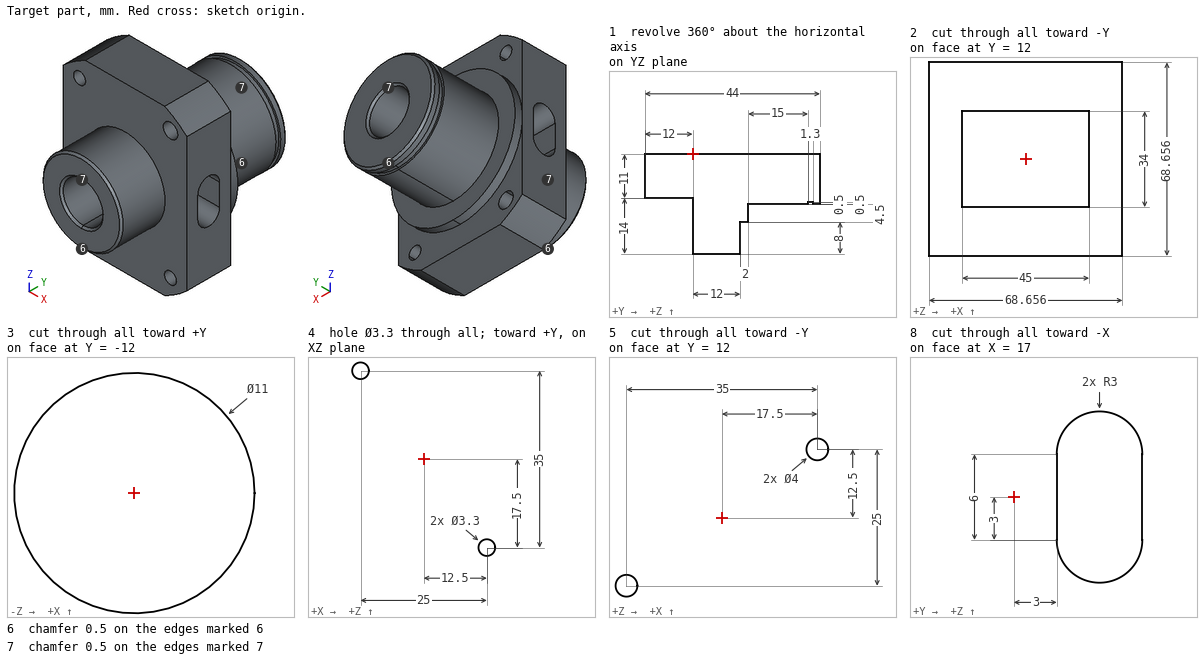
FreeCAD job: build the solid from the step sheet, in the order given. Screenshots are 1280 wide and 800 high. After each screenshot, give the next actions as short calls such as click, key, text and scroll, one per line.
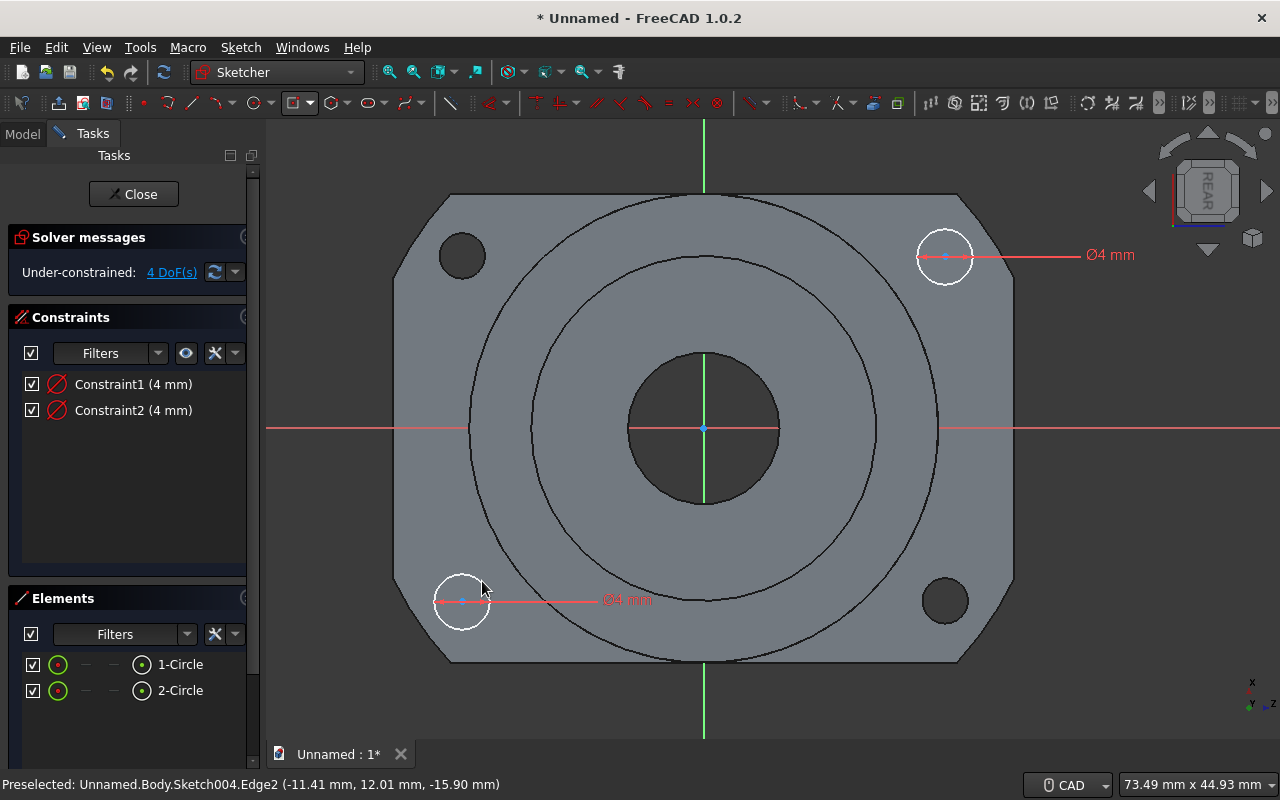
click(490, 104)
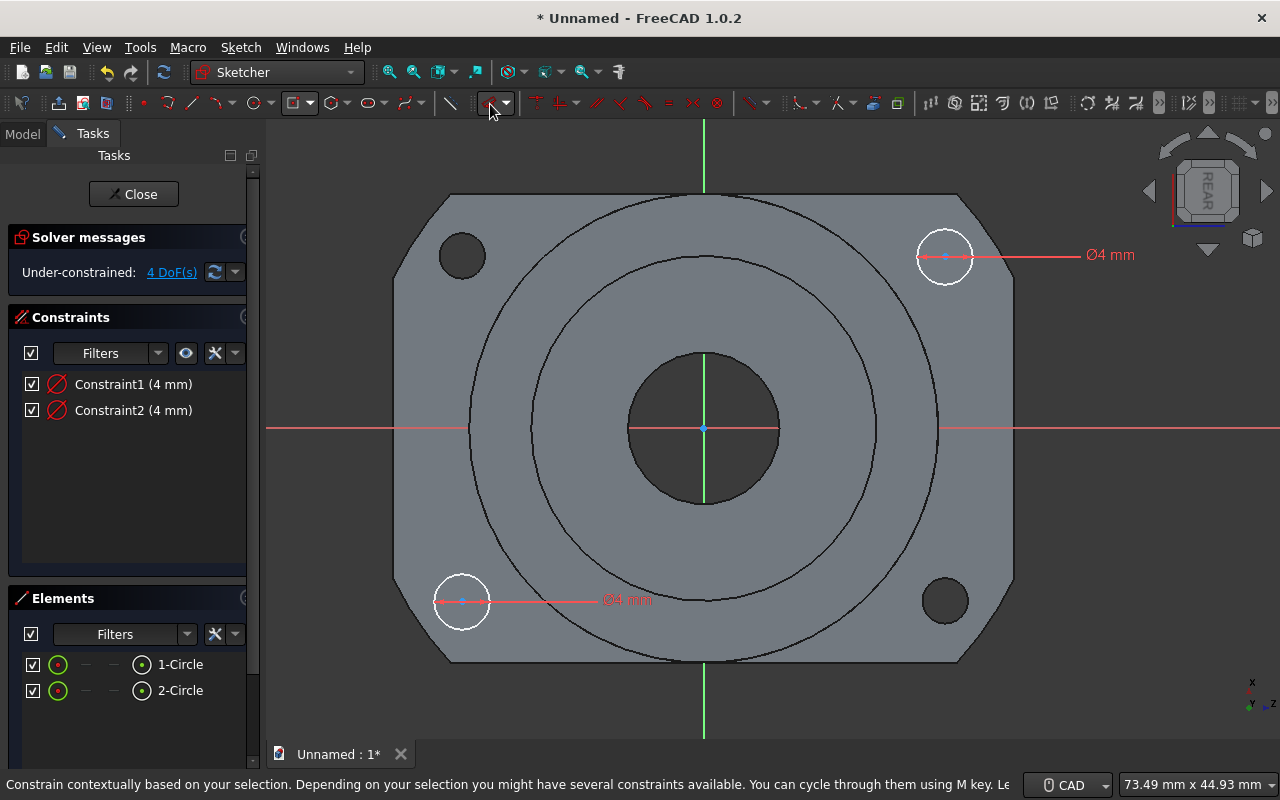
click(945, 257)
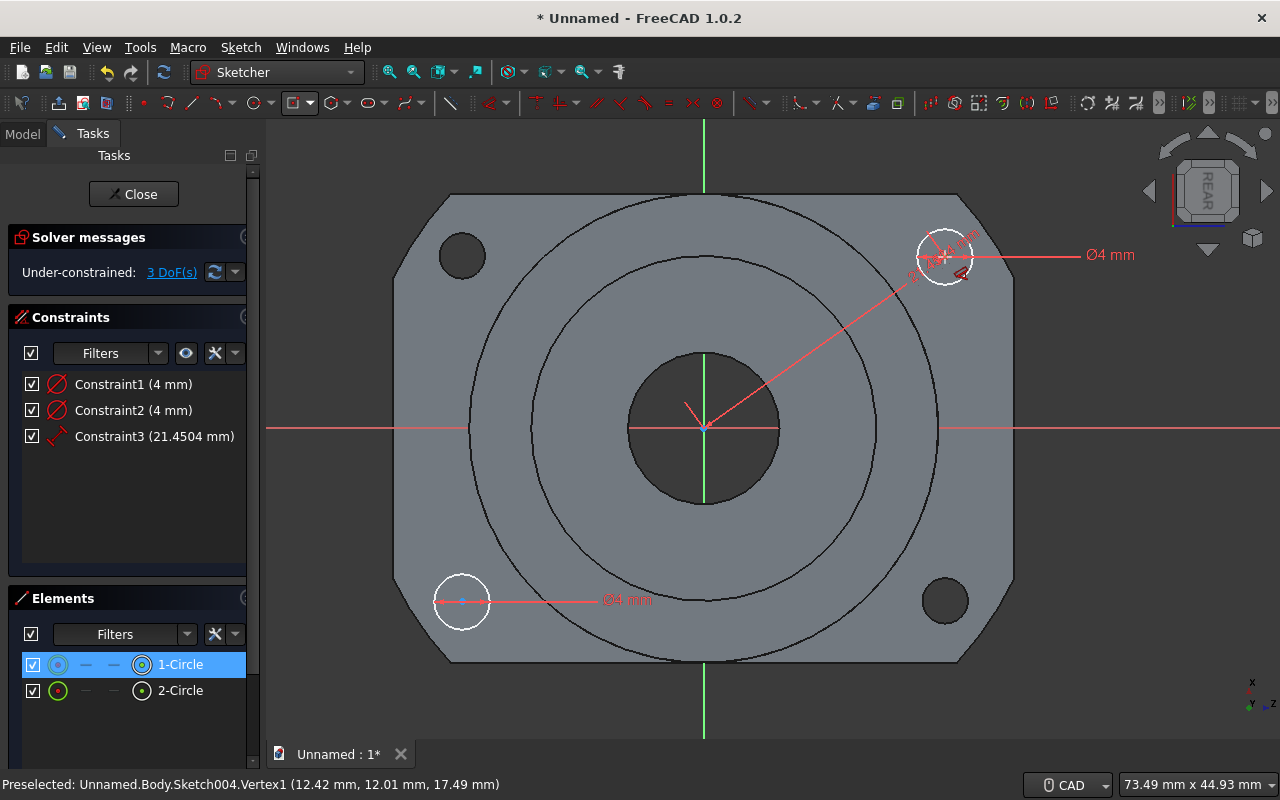
click(462, 602)
click(592, 636)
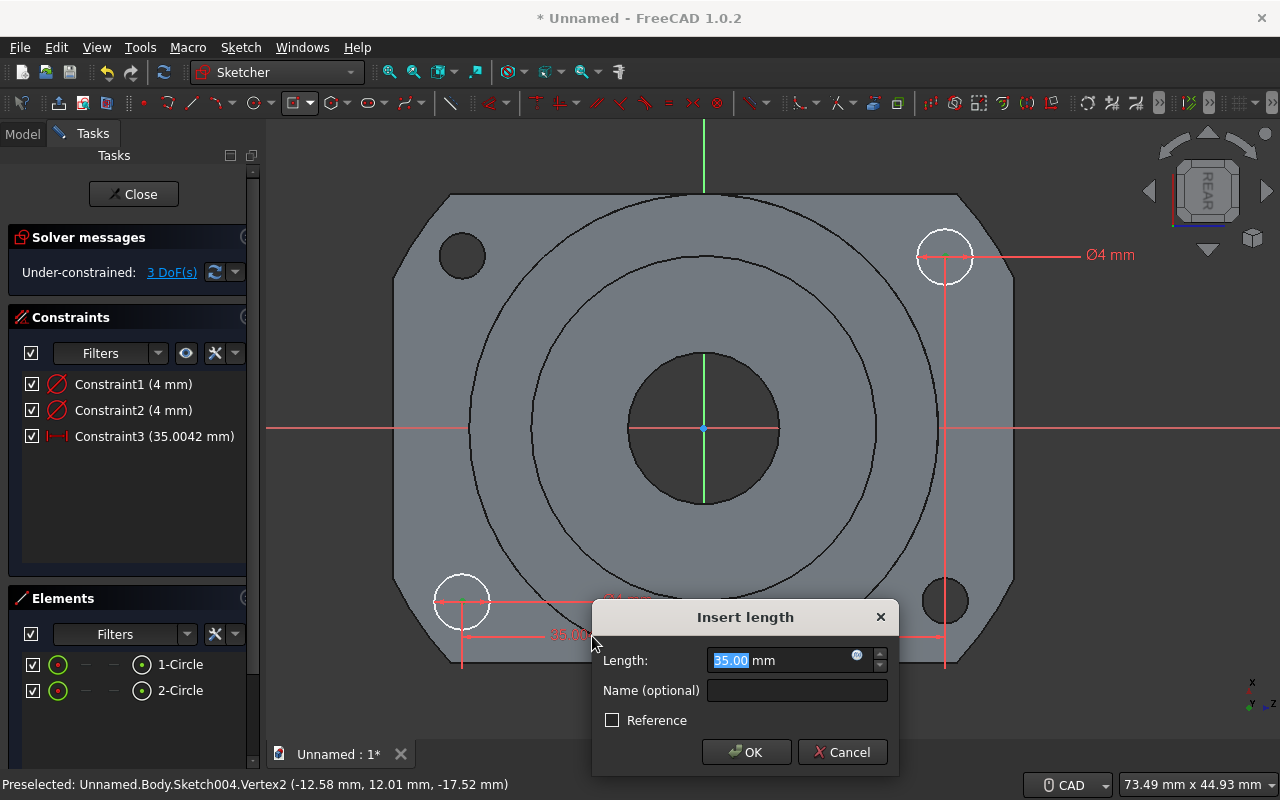
text(35)
key(Return)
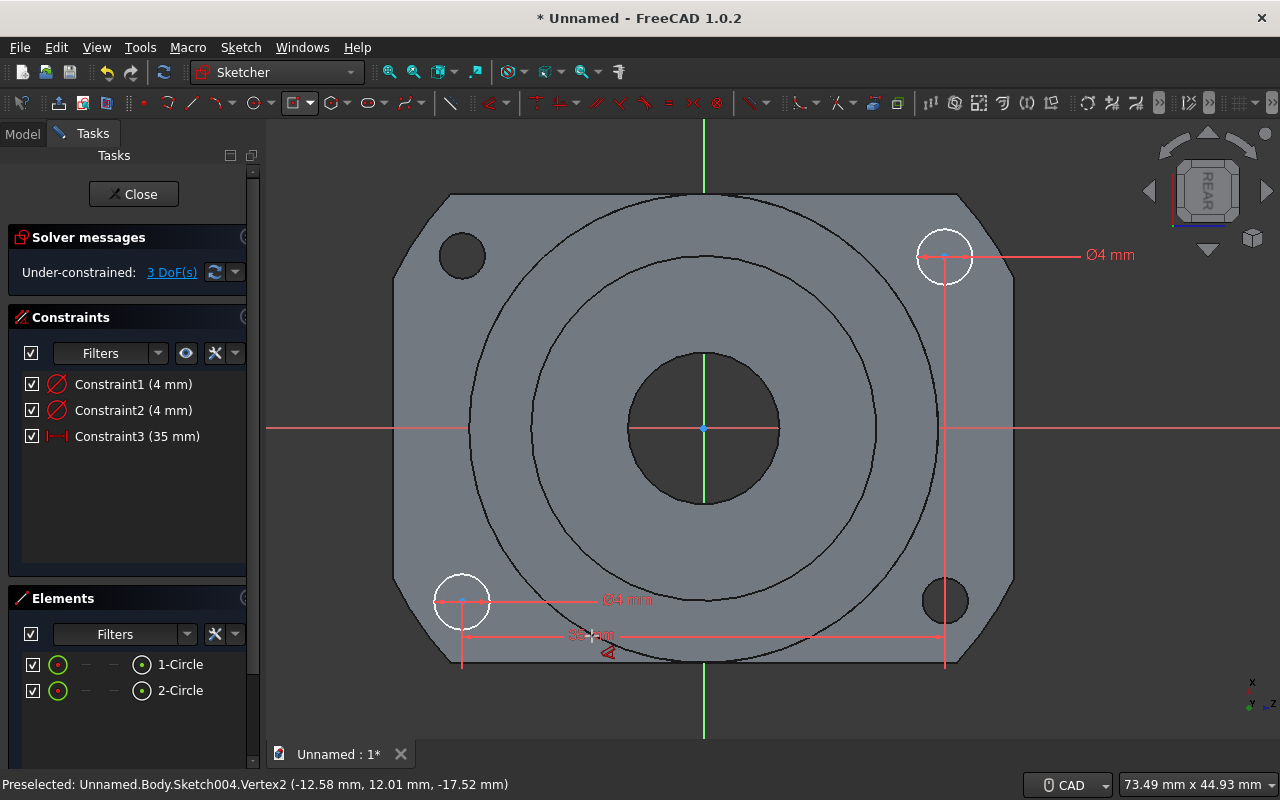
click(945, 257)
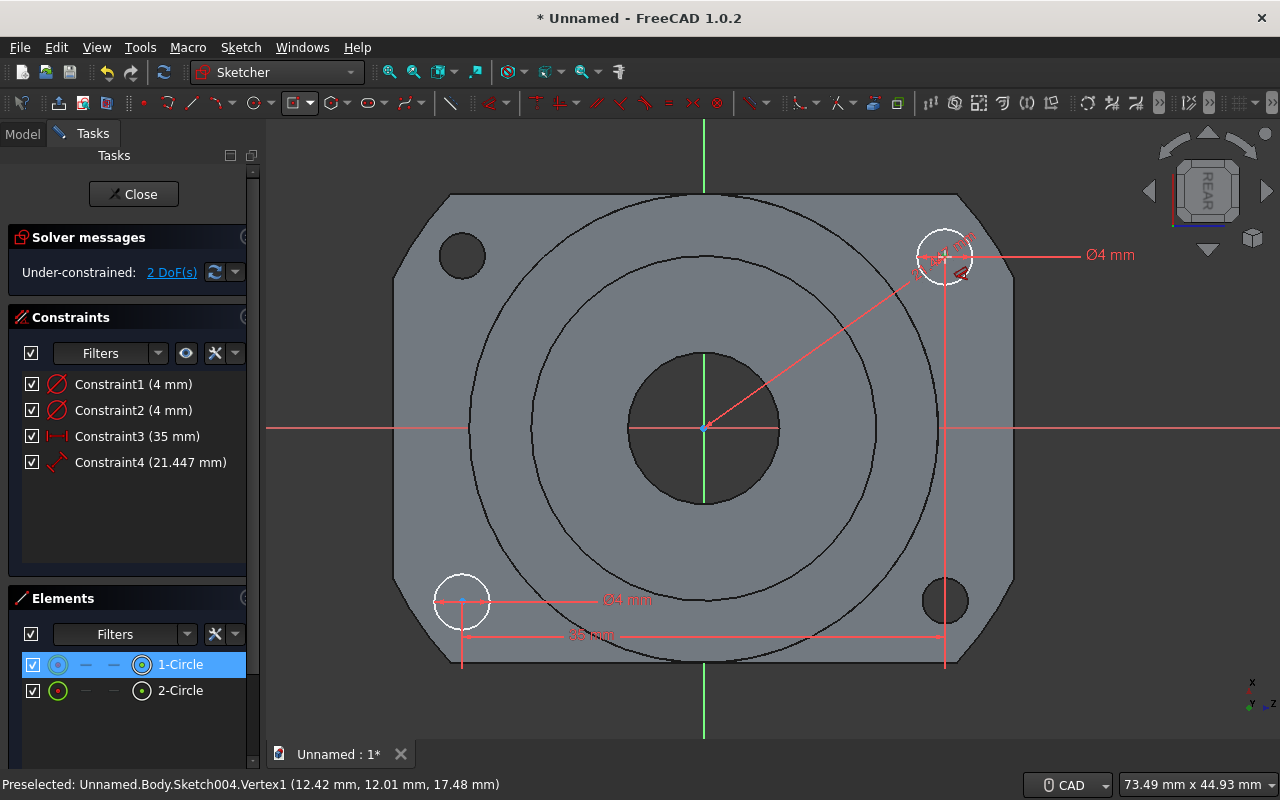
click(462, 602)
click(428, 350)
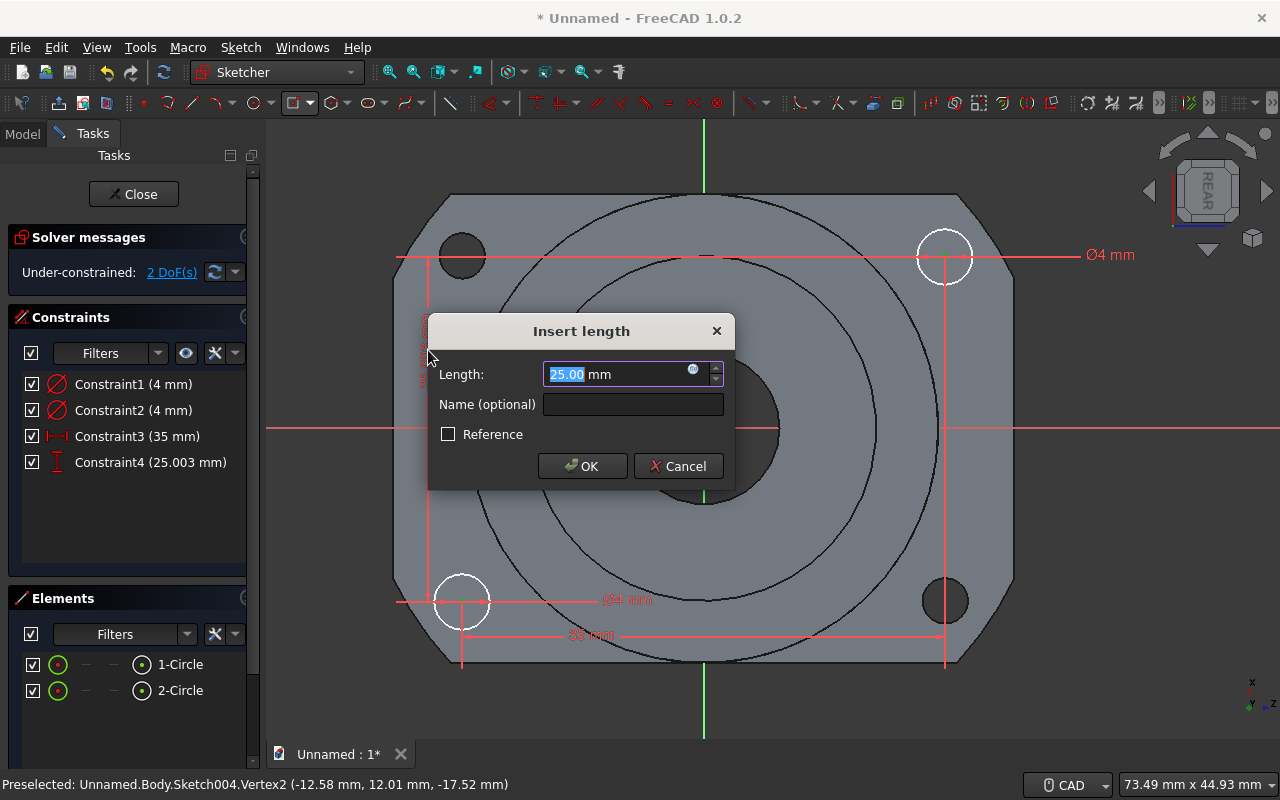
text(25)
key(Return)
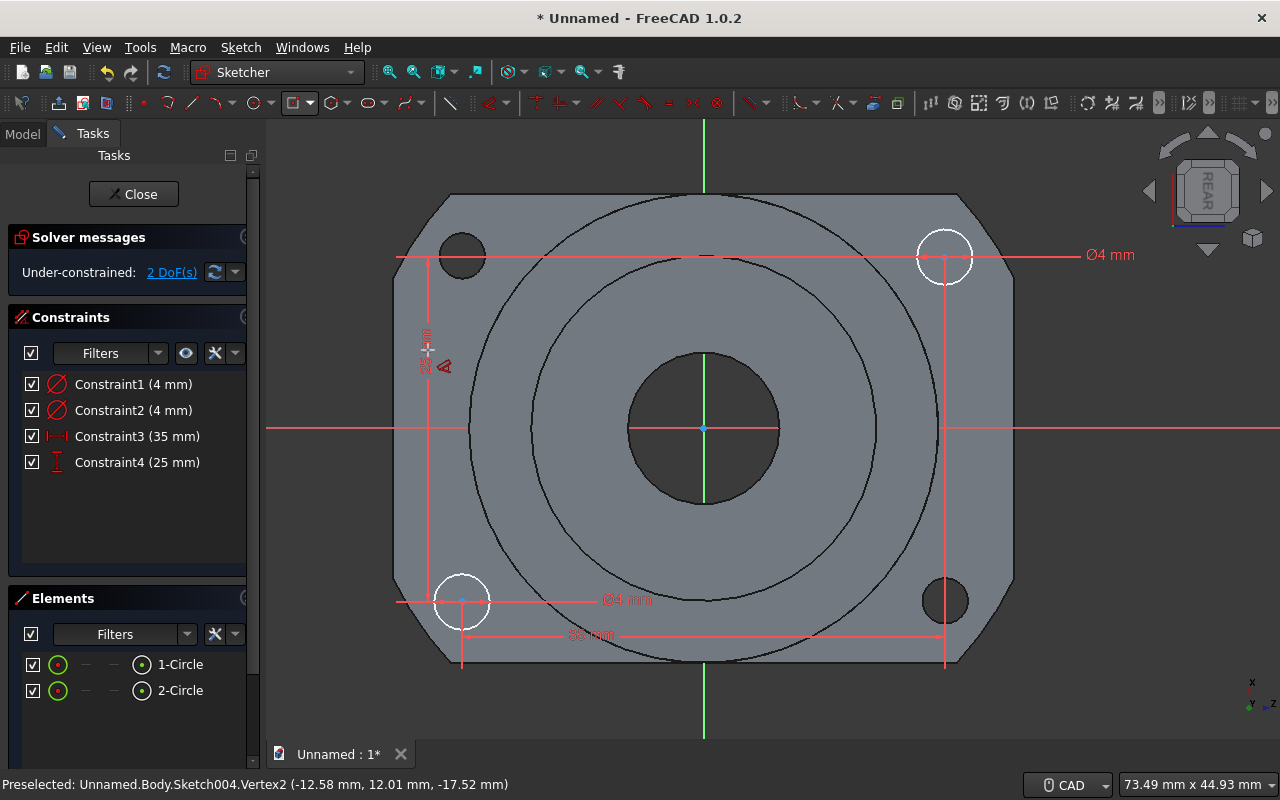
click(945, 257)
click(824, 223)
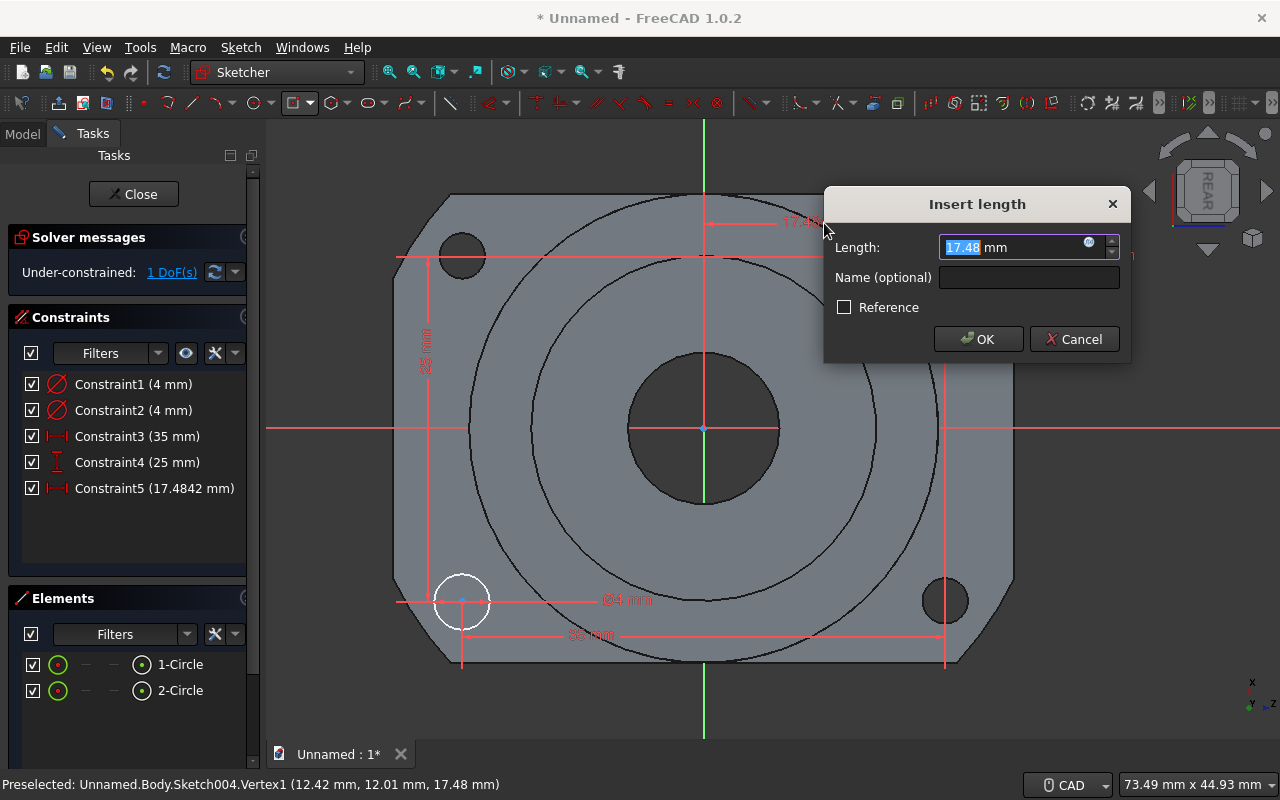
text(17.5)
key(Return)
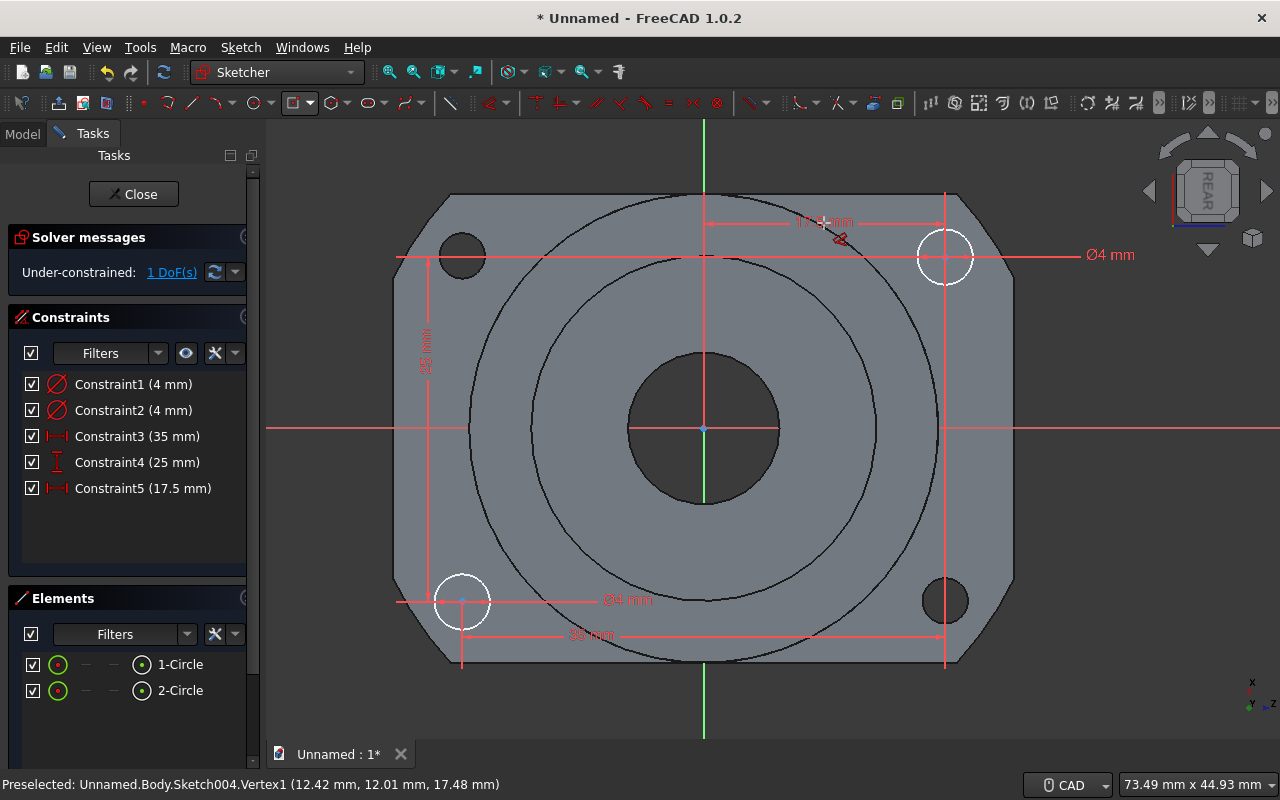
click(945, 257)
click(979, 343)